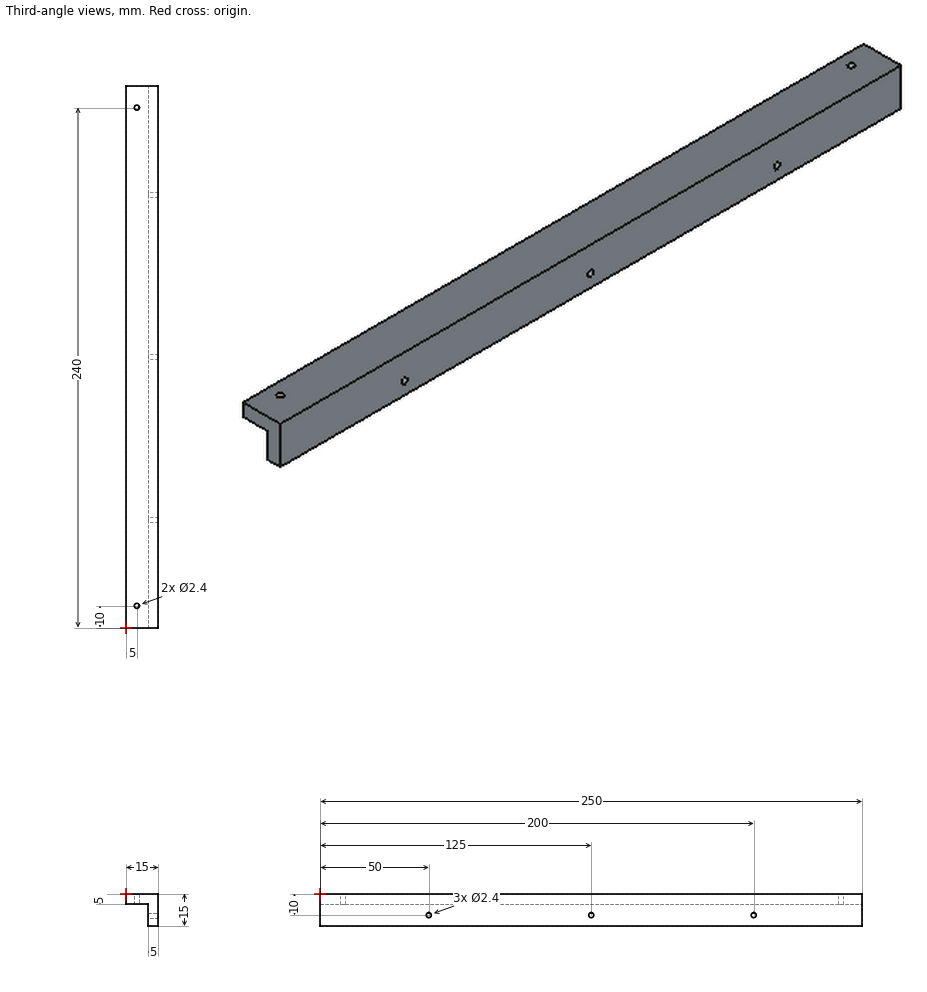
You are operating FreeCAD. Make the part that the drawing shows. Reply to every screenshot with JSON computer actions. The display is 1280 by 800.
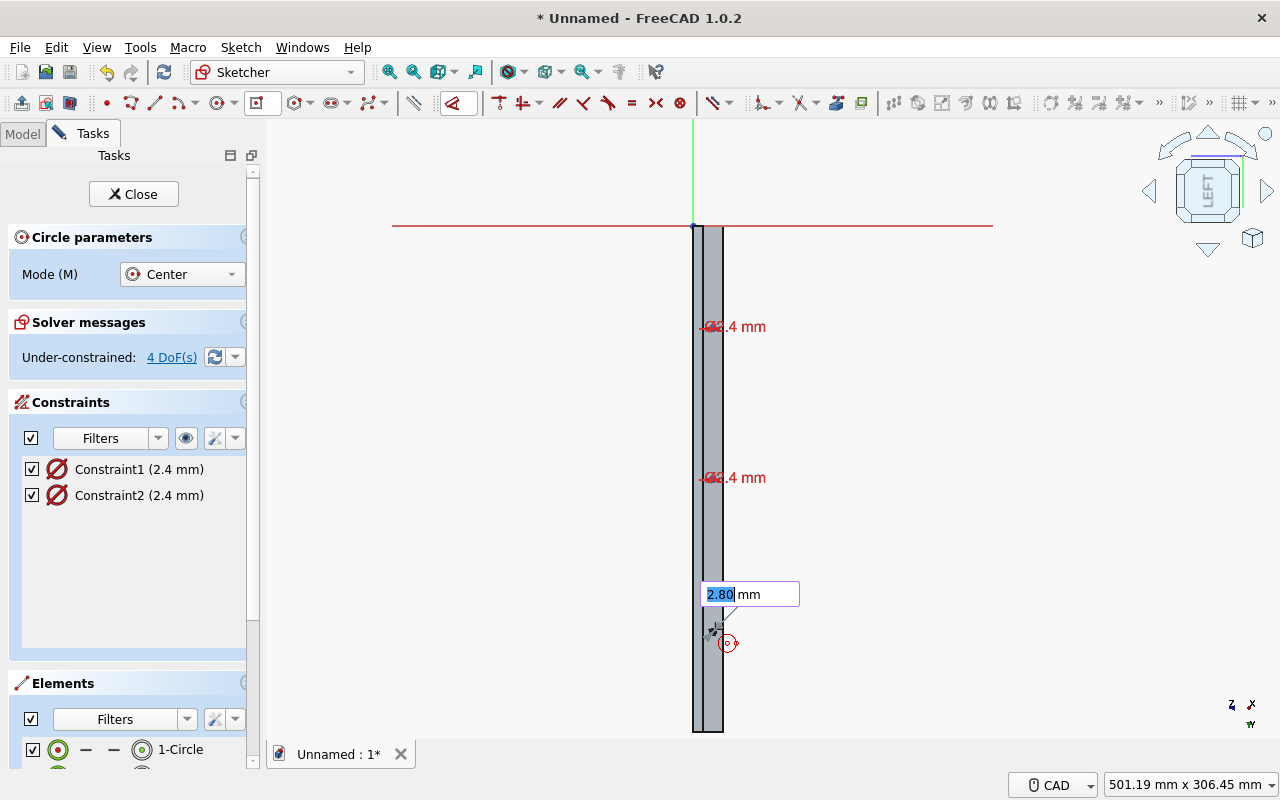
{"action": "type", "text": "2.4"}
{"action": "key", "text": "Return"}
{"action": "key", "text": "Escape"}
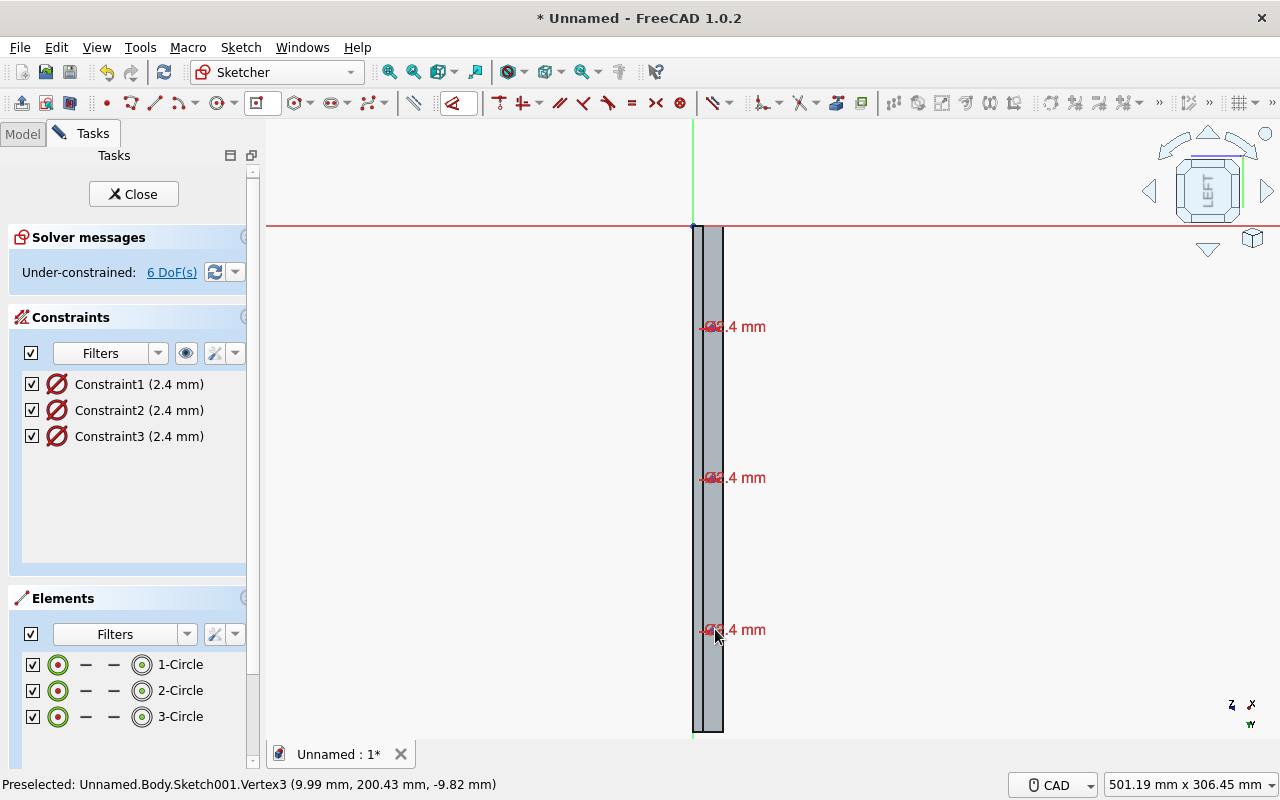
{"action": "key", "text": "d"}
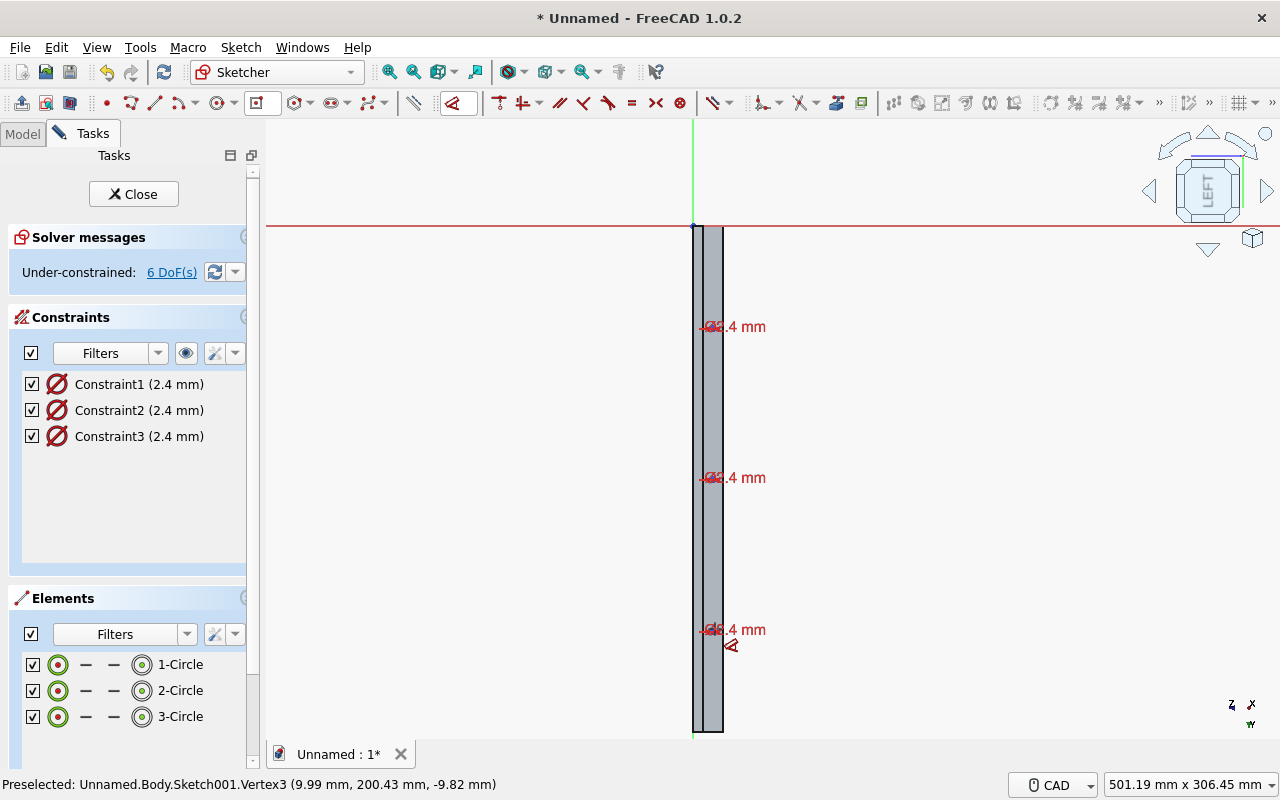
{"action": "scroll", "coordinate": [713, 329], "scroll_direction": "up", "scroll_amount": 4}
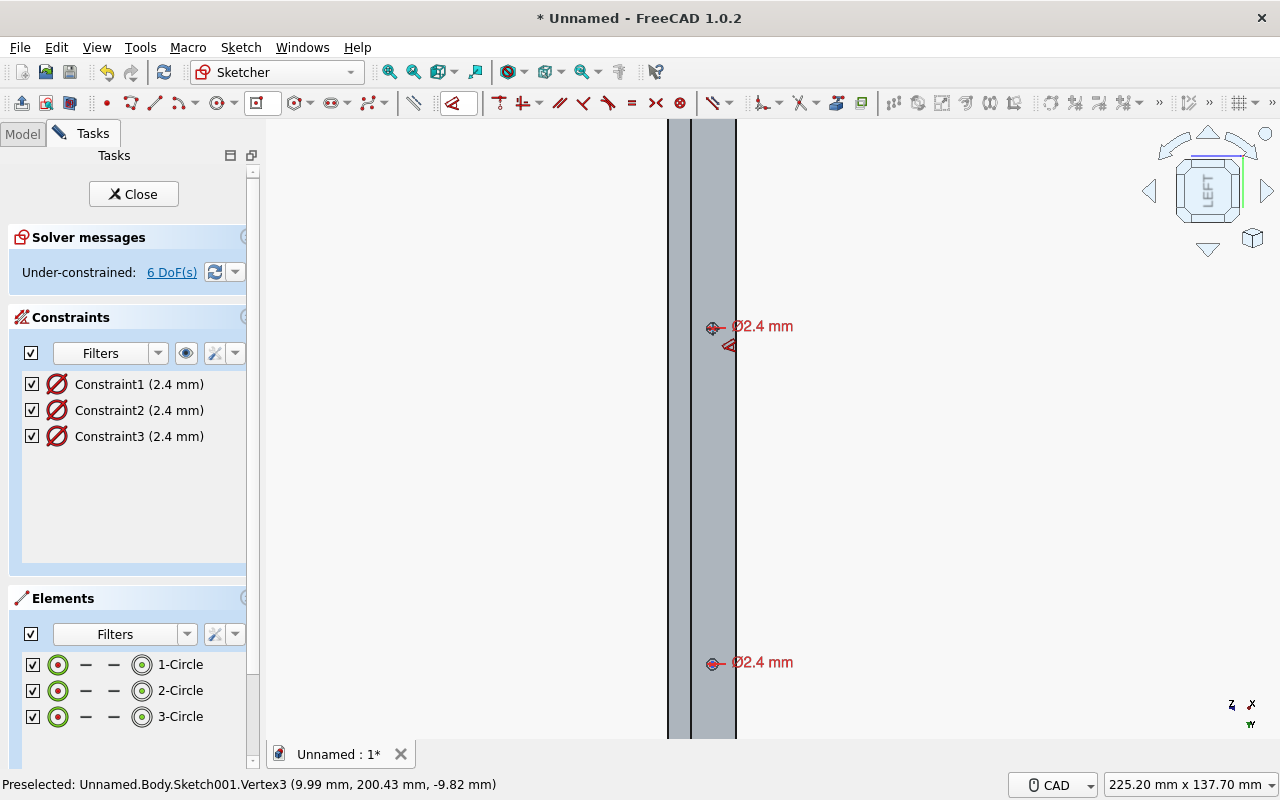
{"action": "left_click", "coordinate": [712, 328]}
{"action": "left_click", "coordinate": [690, 362]}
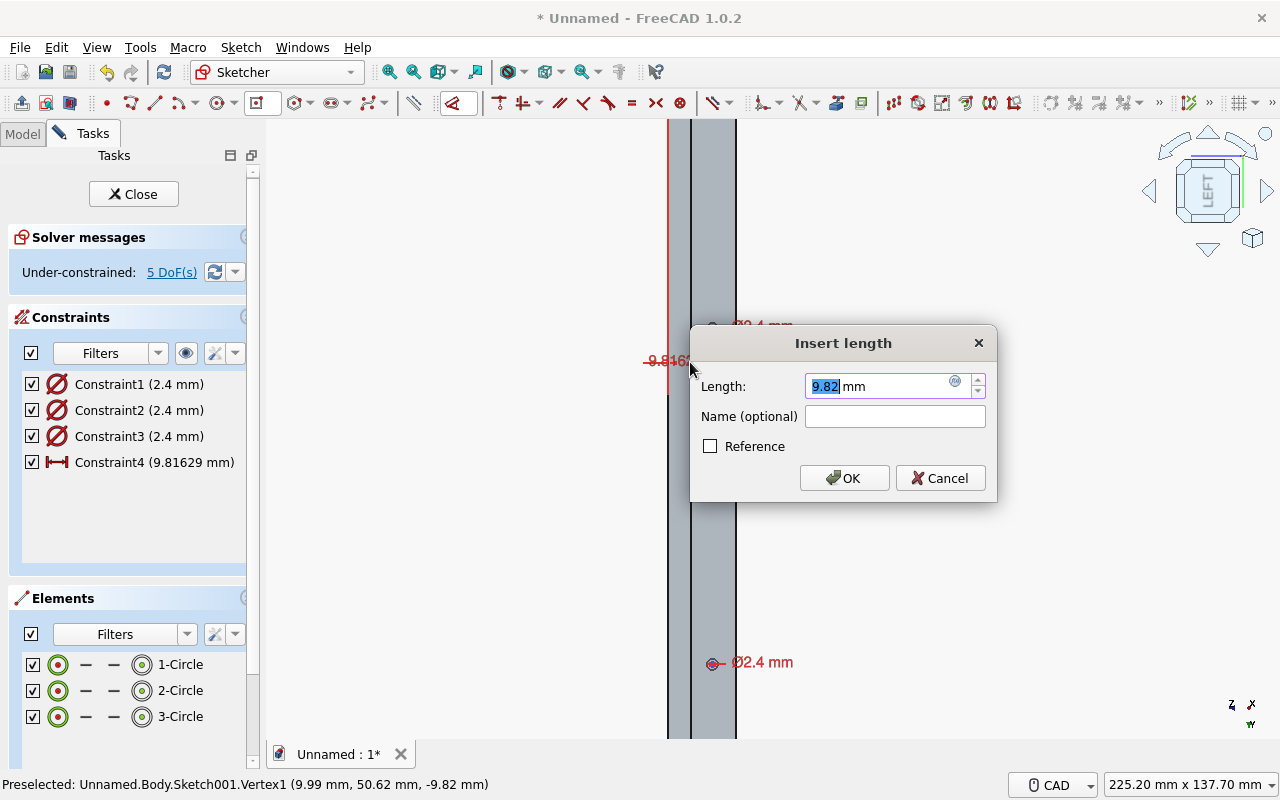
{"action": "type", "text": "10"}
{"action": "key", "text": "Return"}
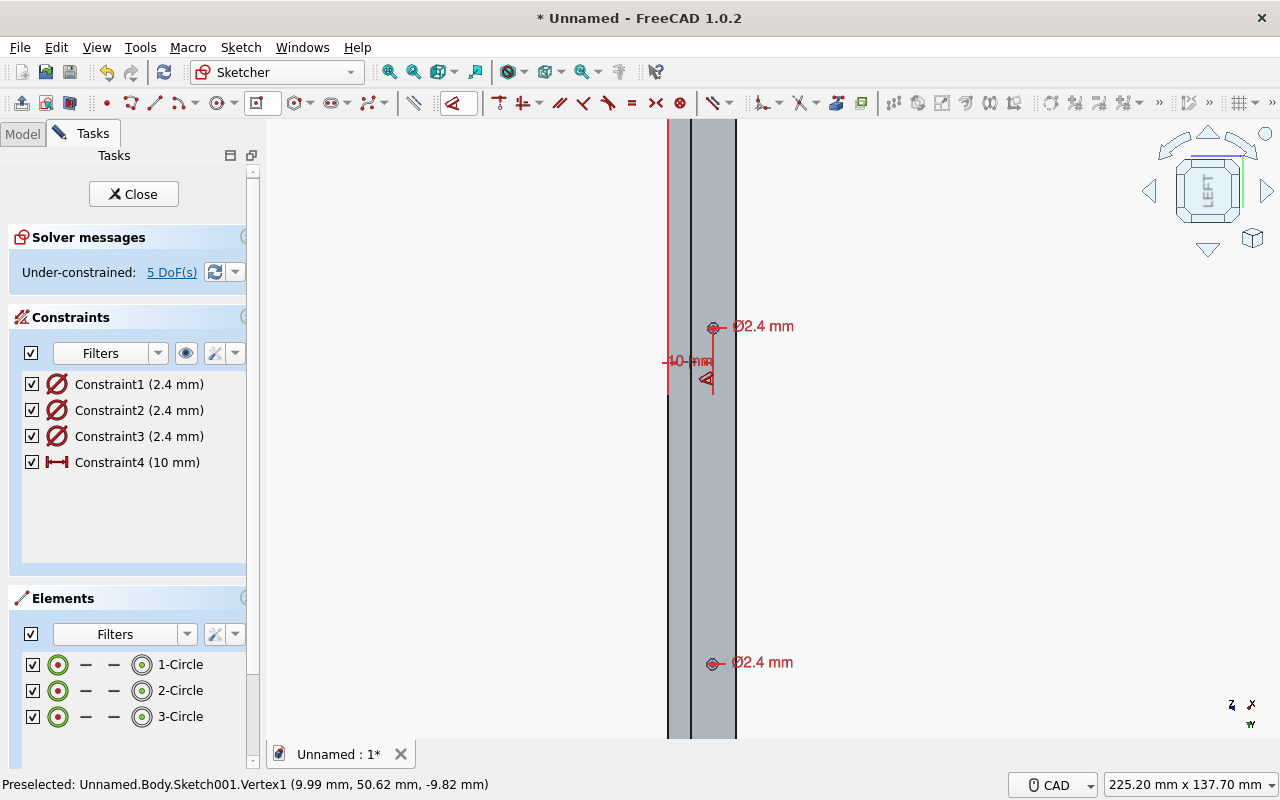
{"action": "left_click", "coordinate": [713, 328]}
{"action": "left_click", "coordinate": [634, 238]}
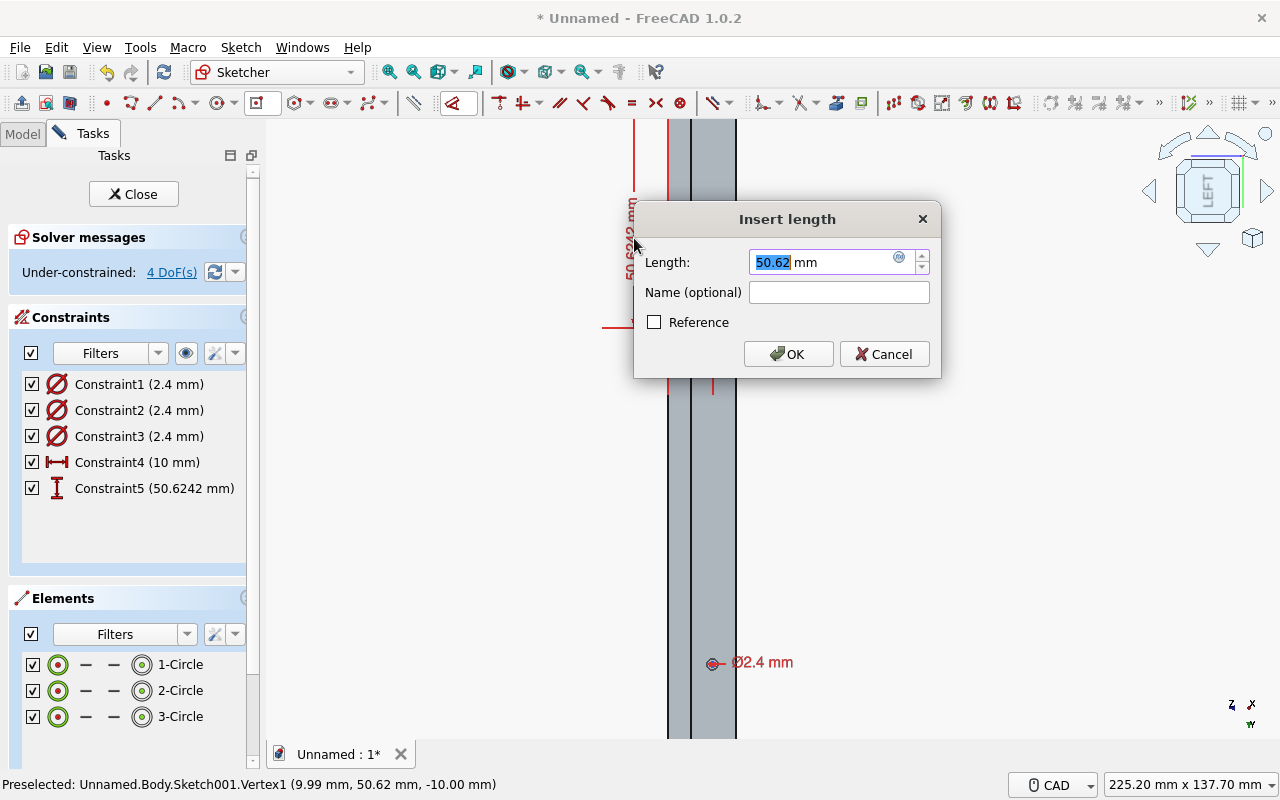
{"action": "type", "text": "50"}
{"action": "key", "text": "Return"}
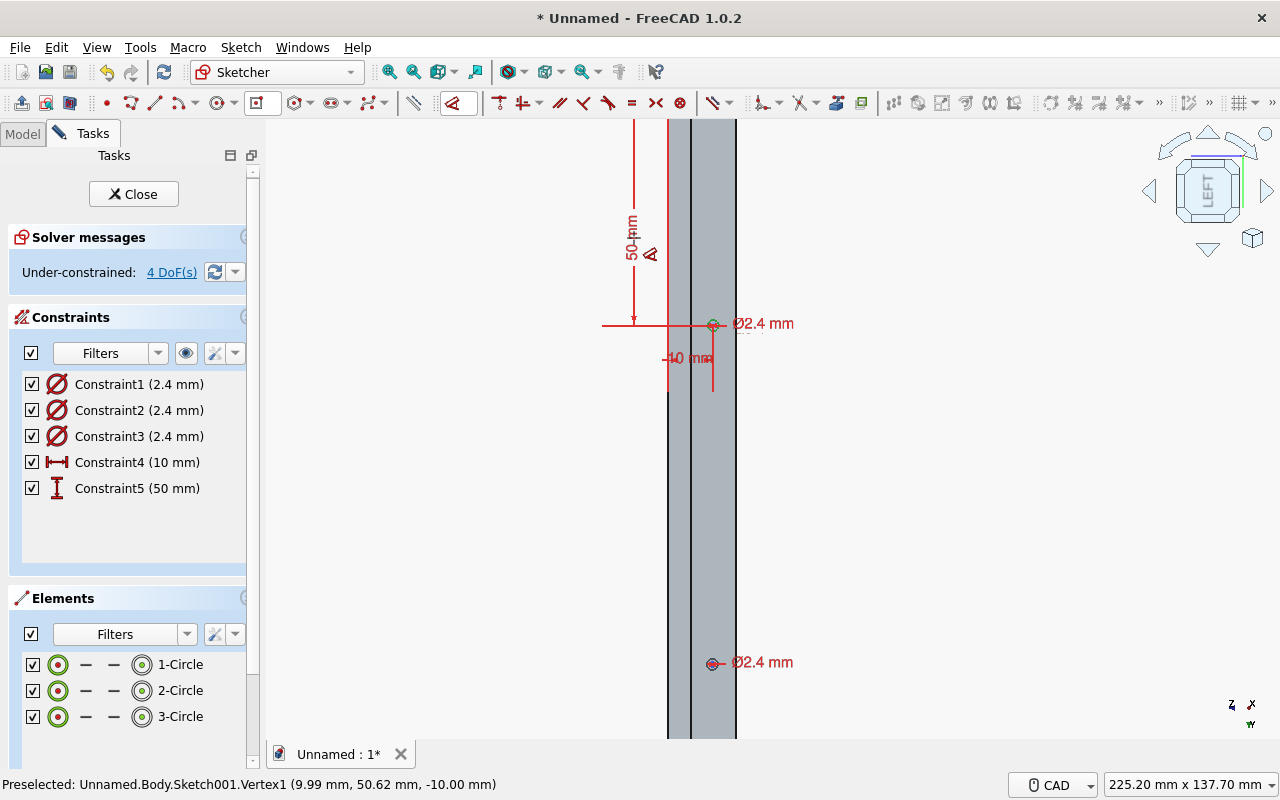
{"action": "left_click", "coordinate": [712, 664]}
{"action": "left_click", "coordinate": [690, 698]}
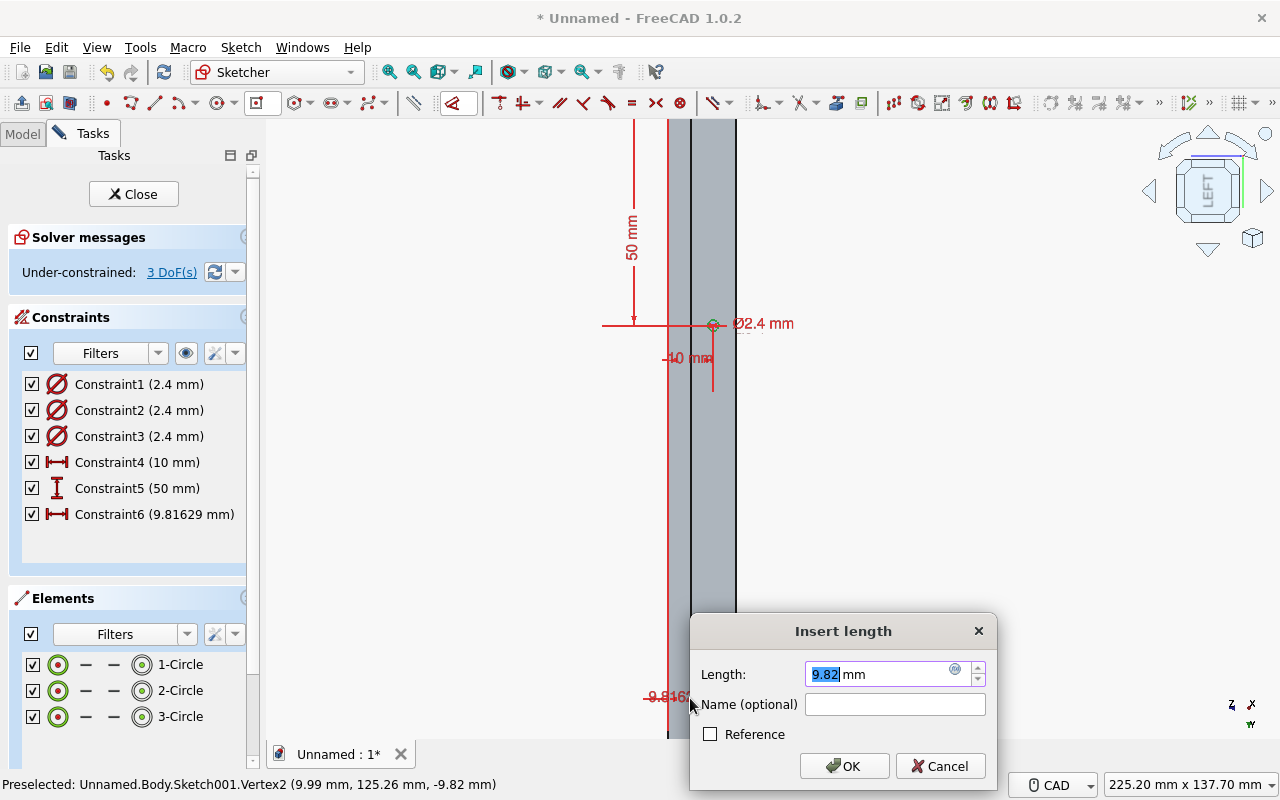
{"action": "type", "text": "10"}
{"action": "key", "text": "Return"}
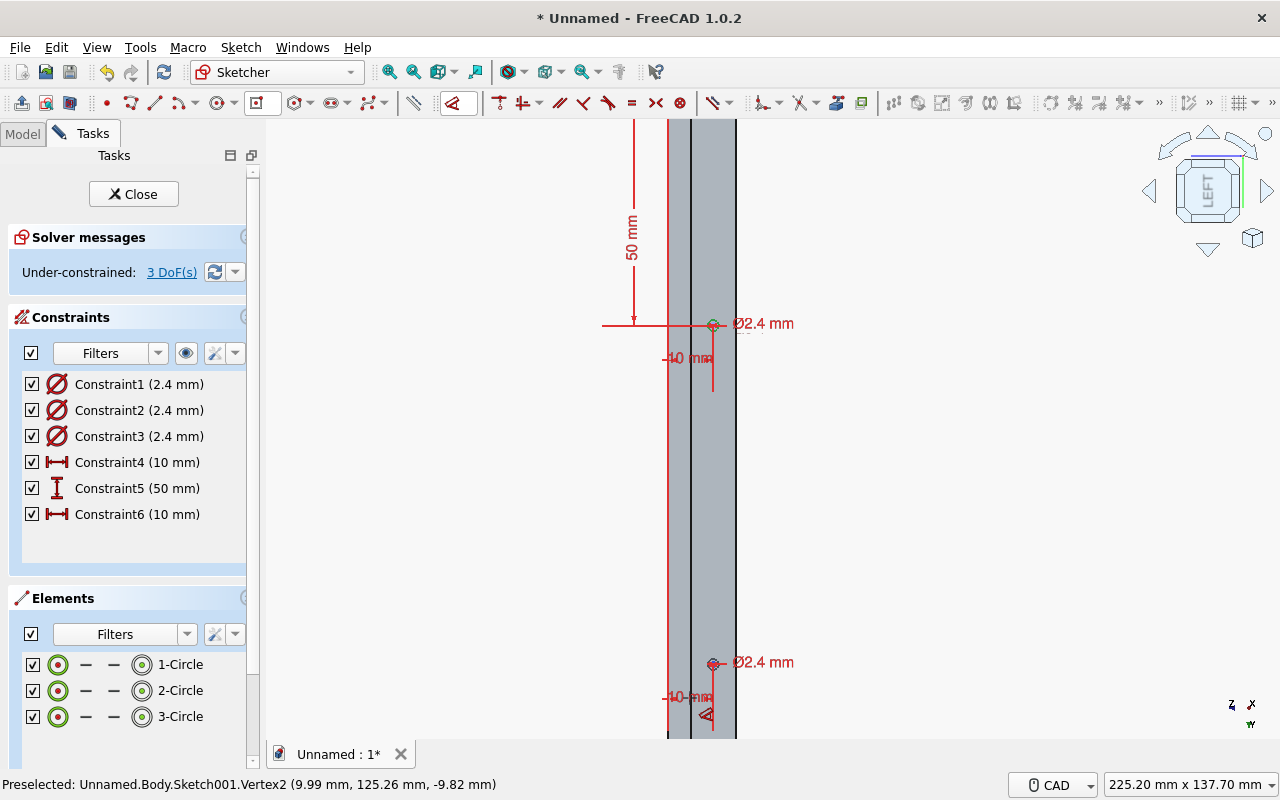
{"action": "scroll", "coordinate": [713, 327], "scroll_direction": "down", "scroll_amount": 4}